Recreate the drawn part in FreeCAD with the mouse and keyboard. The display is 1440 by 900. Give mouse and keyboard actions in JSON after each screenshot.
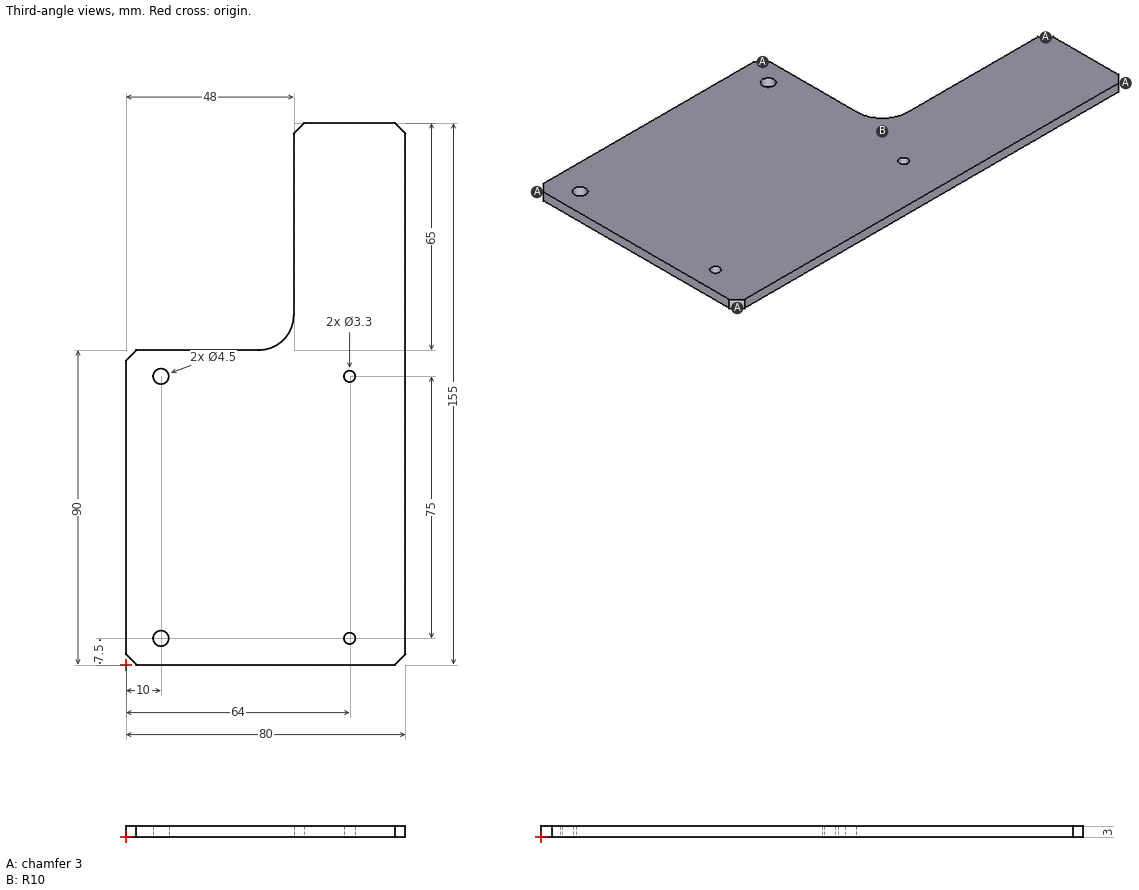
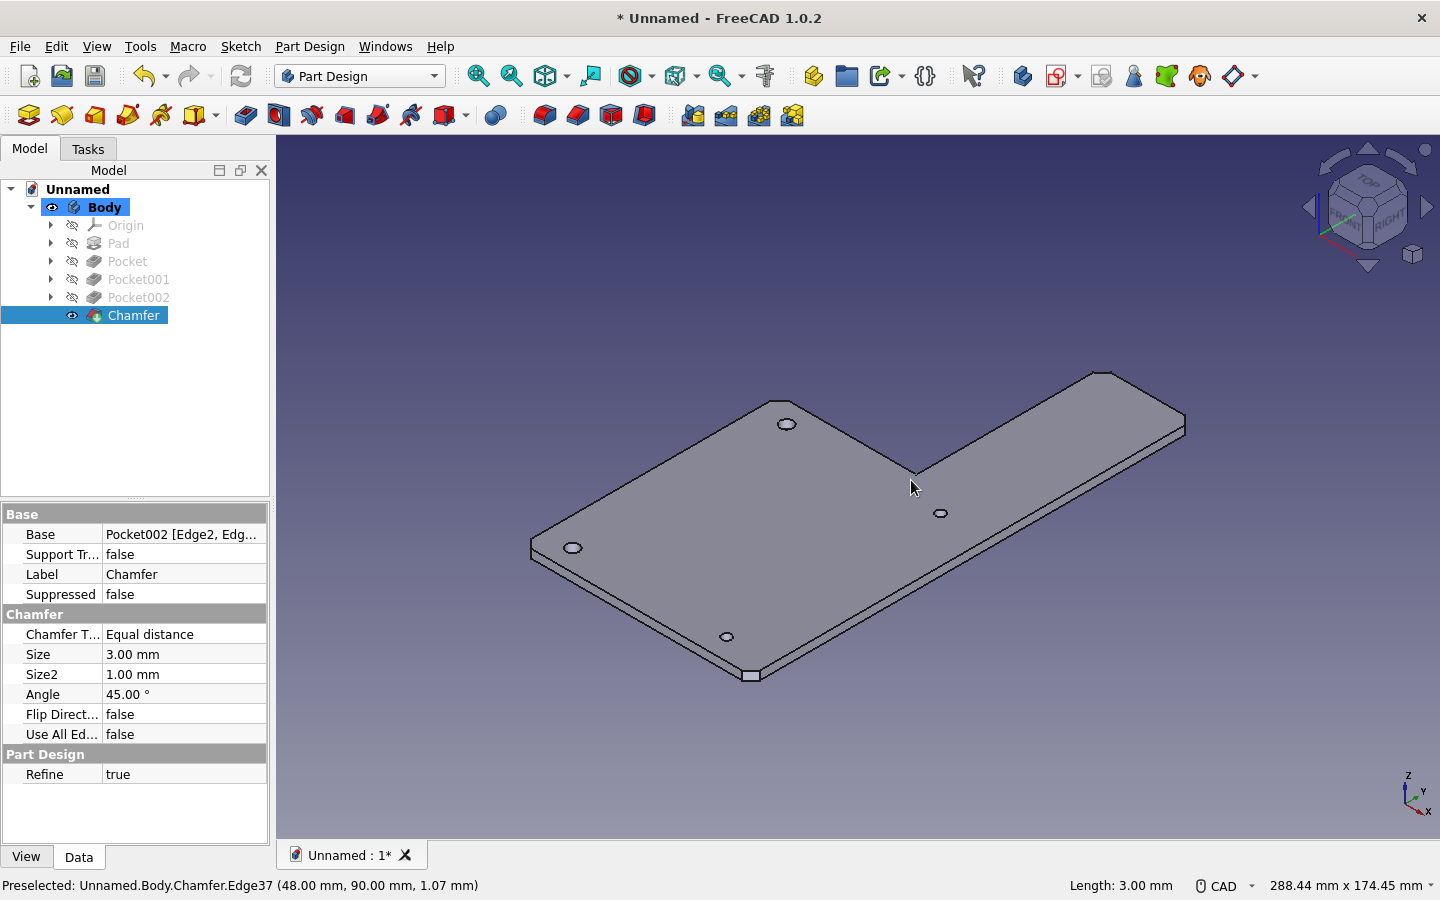
{"action": "left_click", "coordinate": [545, 116]}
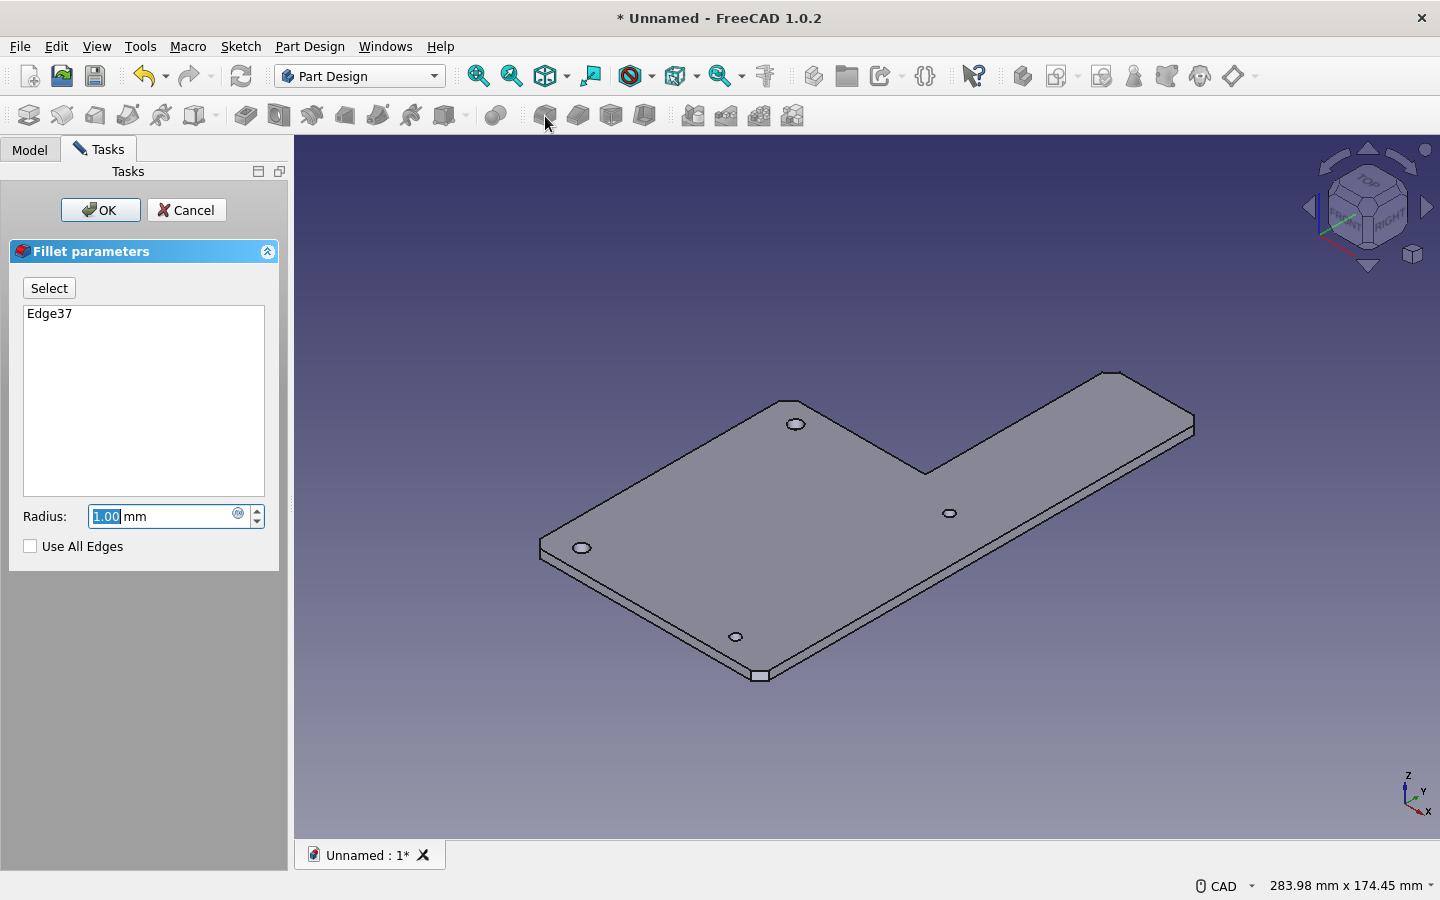
{"action": "type", "text": "10"}
{"action": "key", "text": "Tab"}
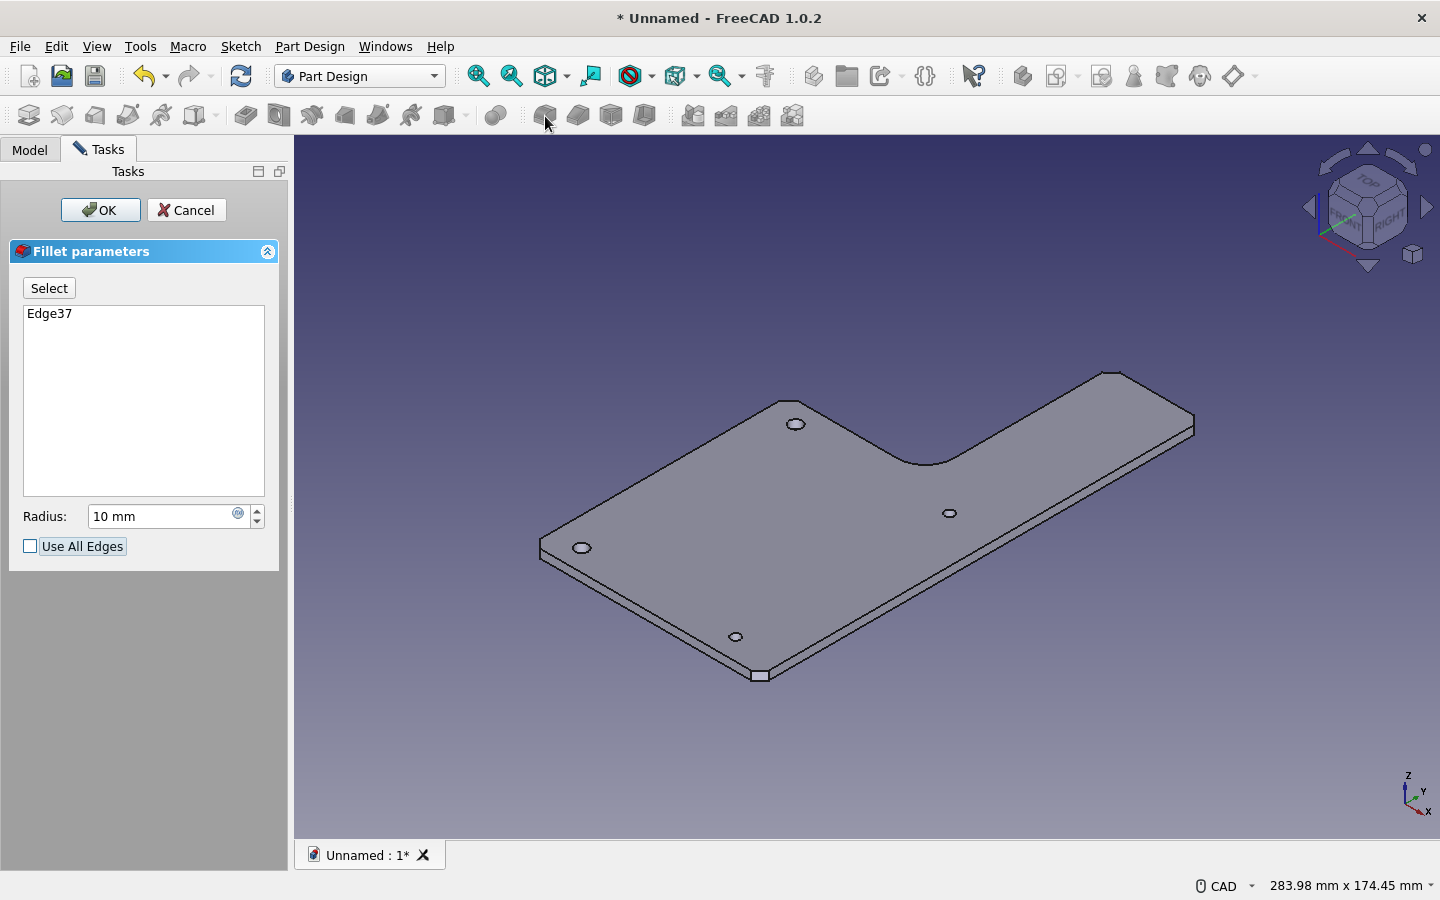
{"action": "left_click", "coordinate": [101, 210]}